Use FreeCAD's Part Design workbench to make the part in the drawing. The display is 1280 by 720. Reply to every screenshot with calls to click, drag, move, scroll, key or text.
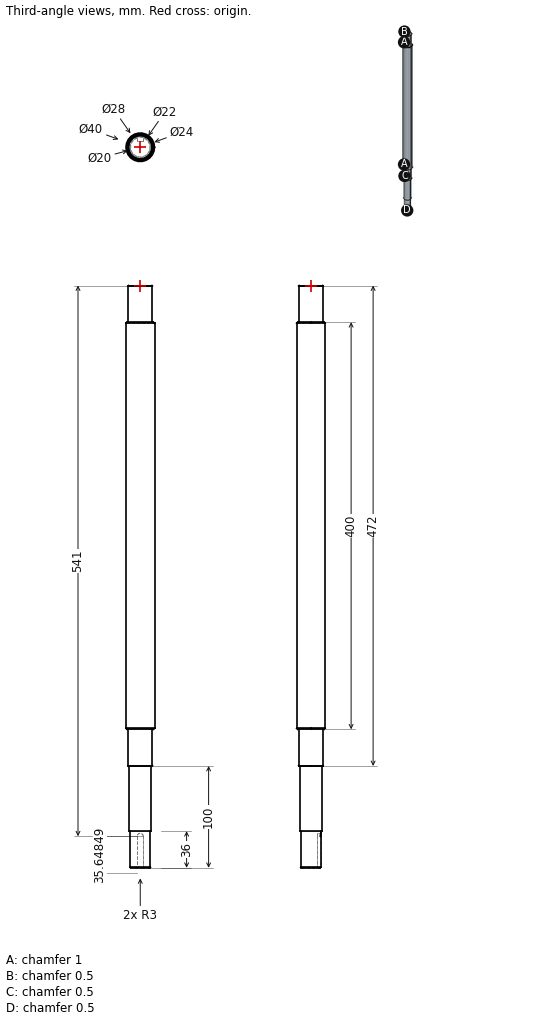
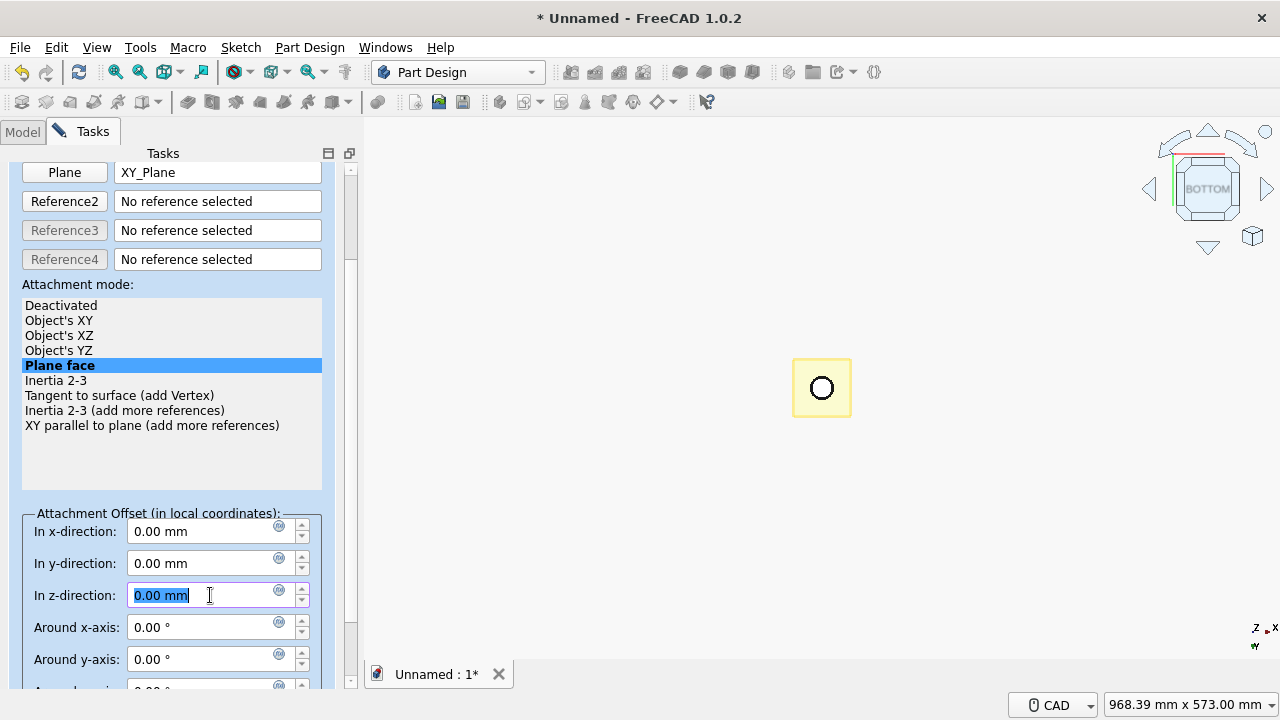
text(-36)
key(Tab)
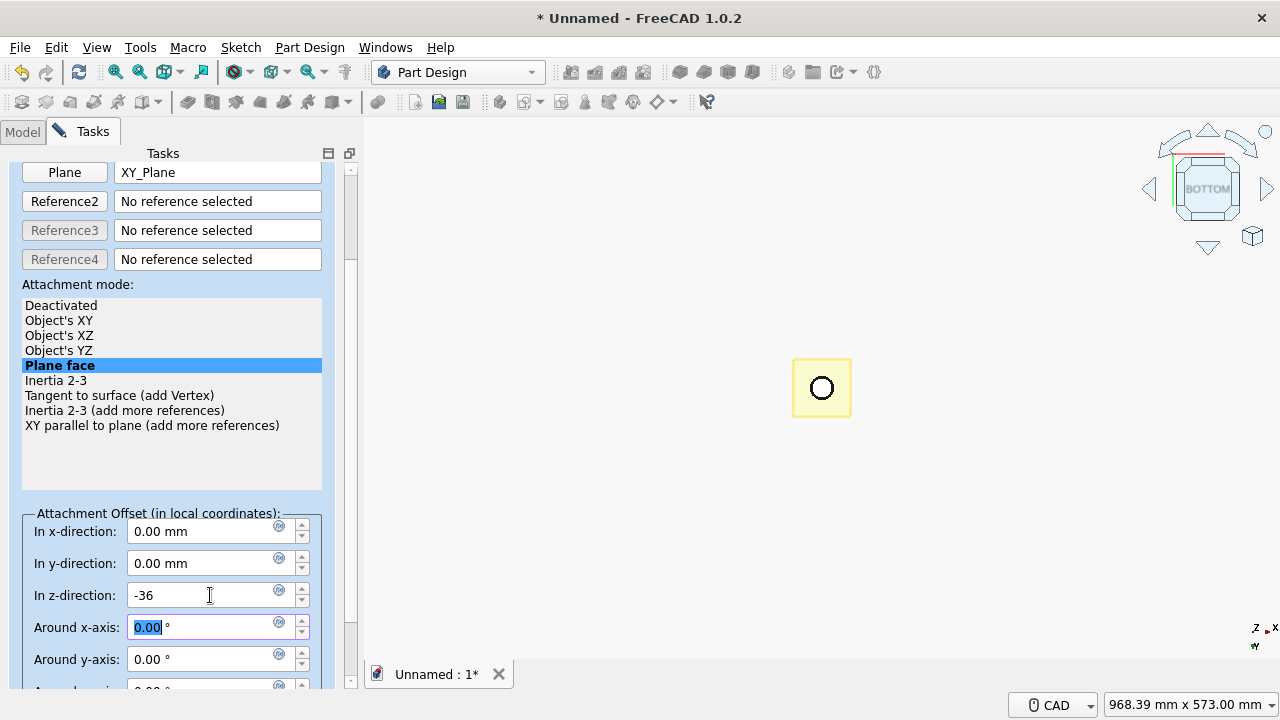
scroll(351, 426, up, 3)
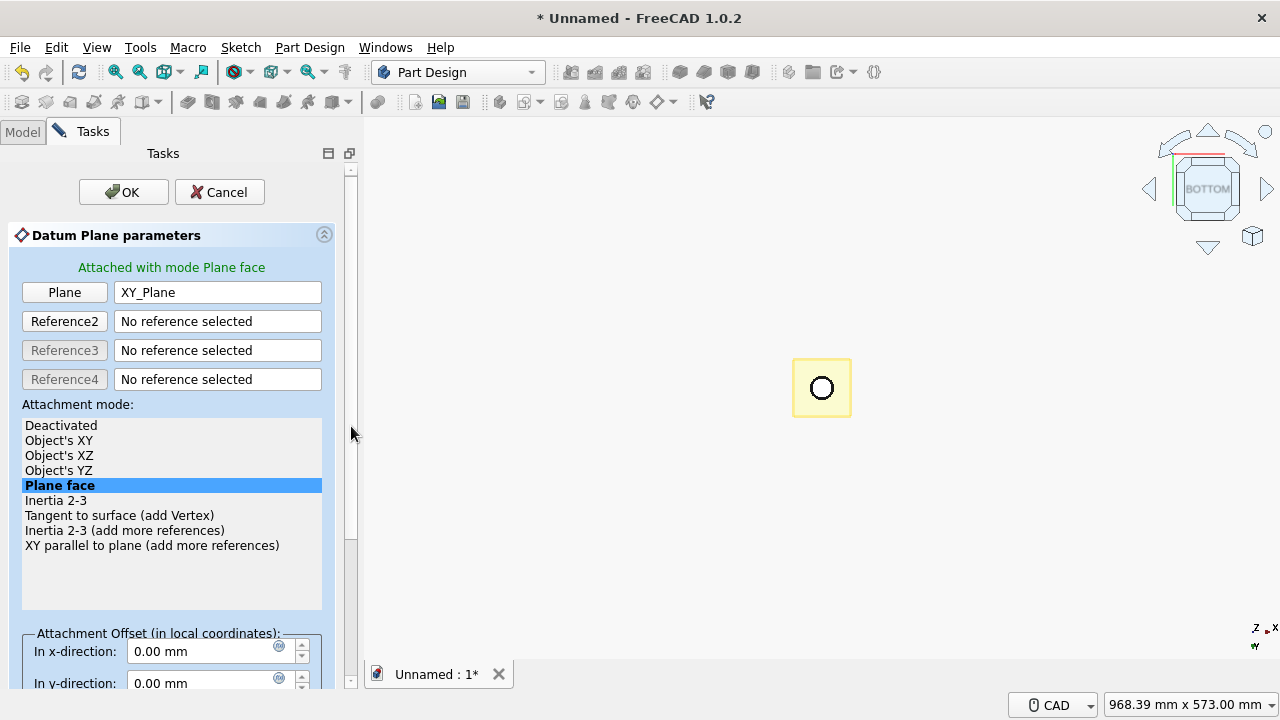
click(124, 192)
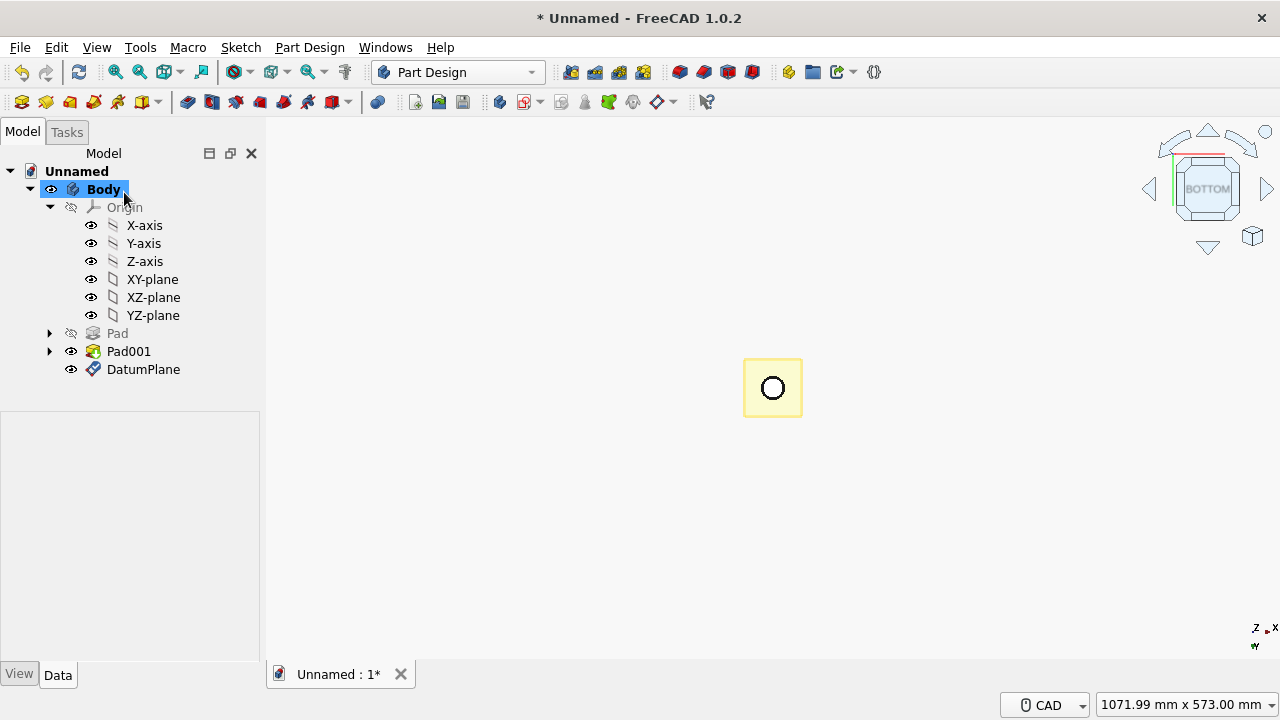
click(116, 369)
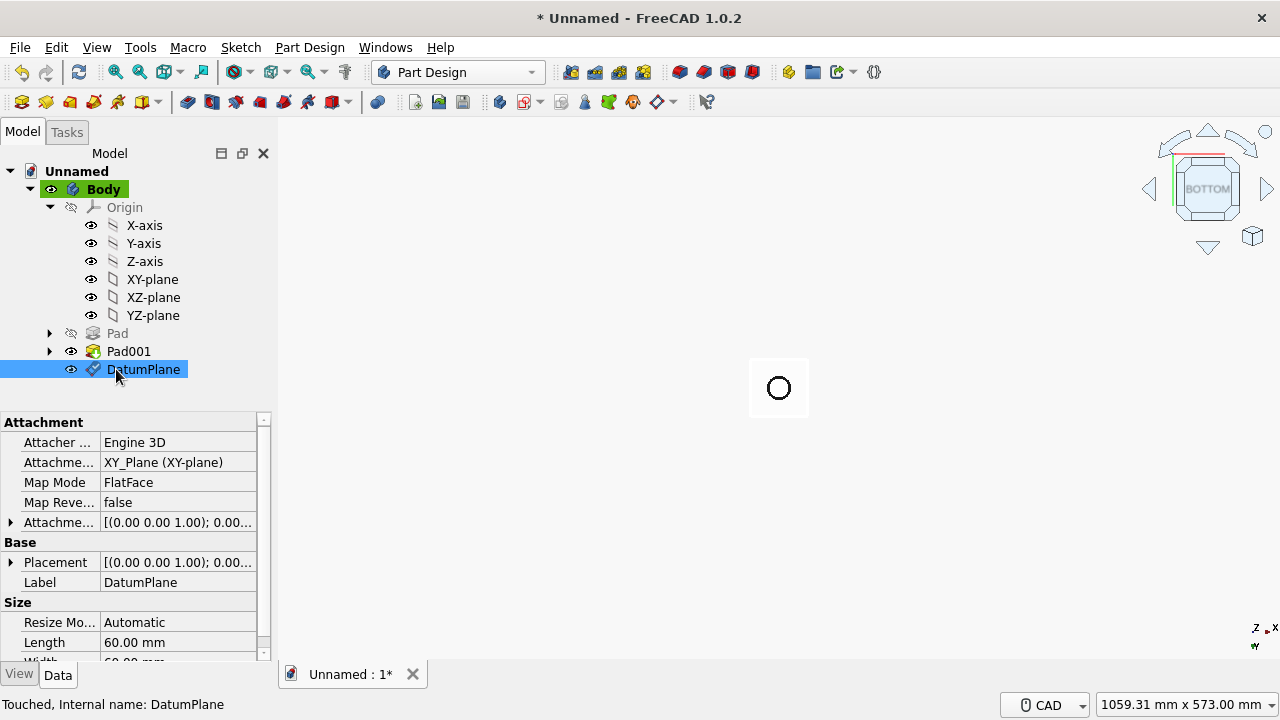
click(524, 102)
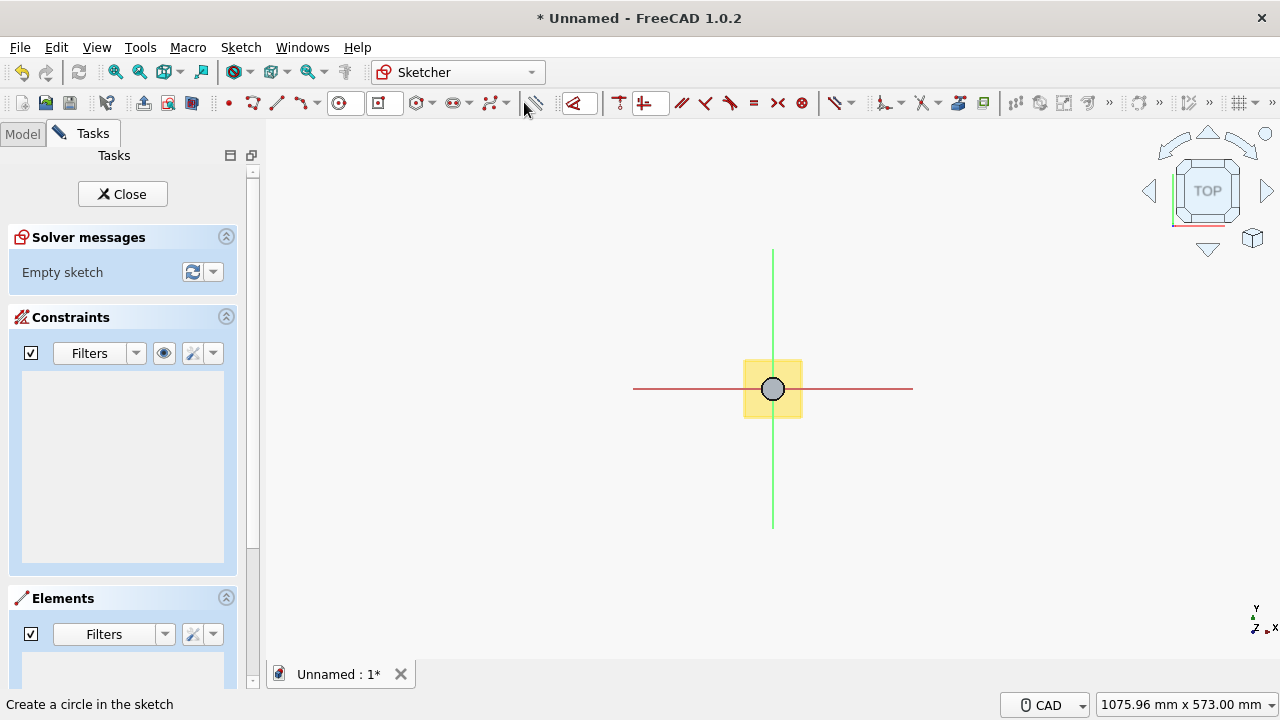
click(192, 104)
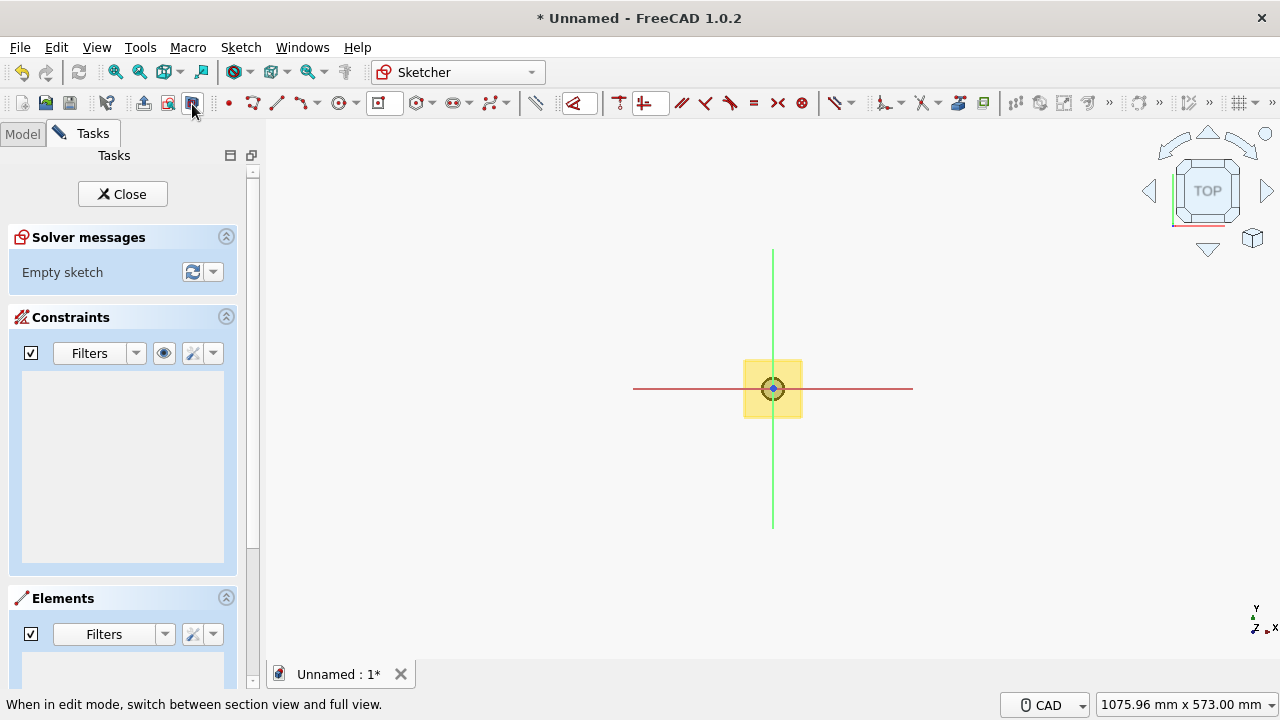
scroll(778, 389, up, 13)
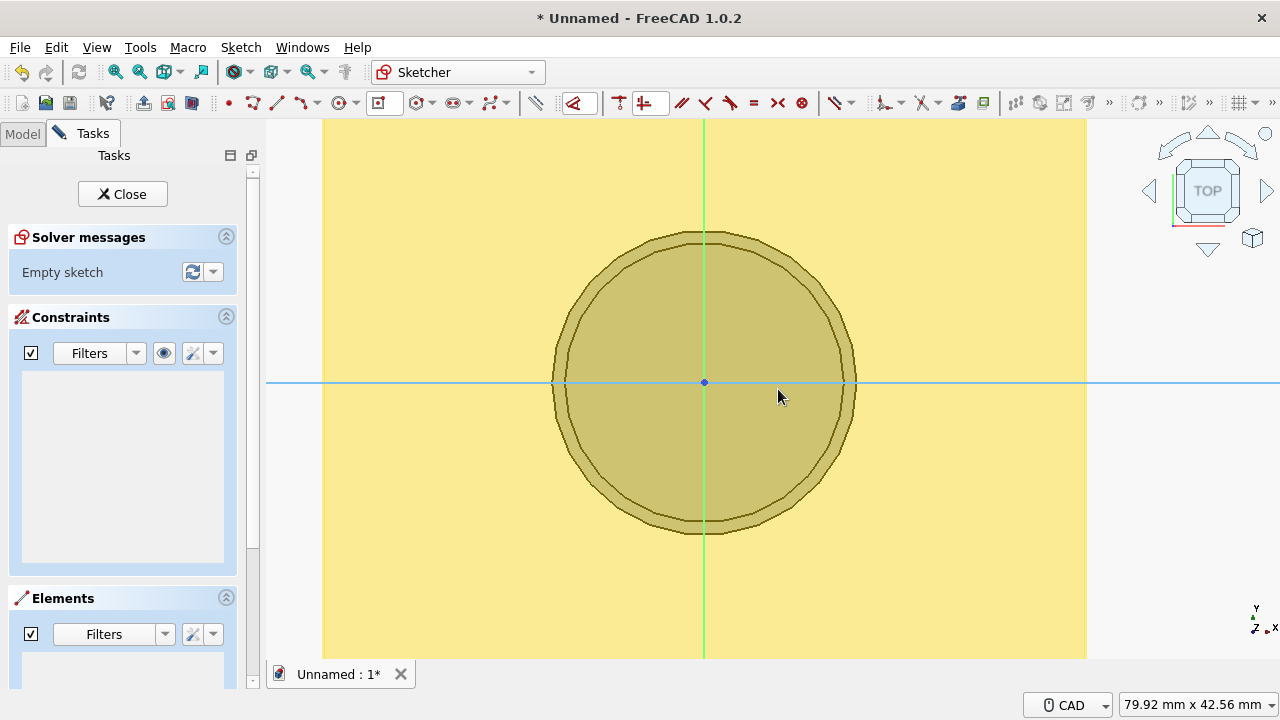
click(340, 104)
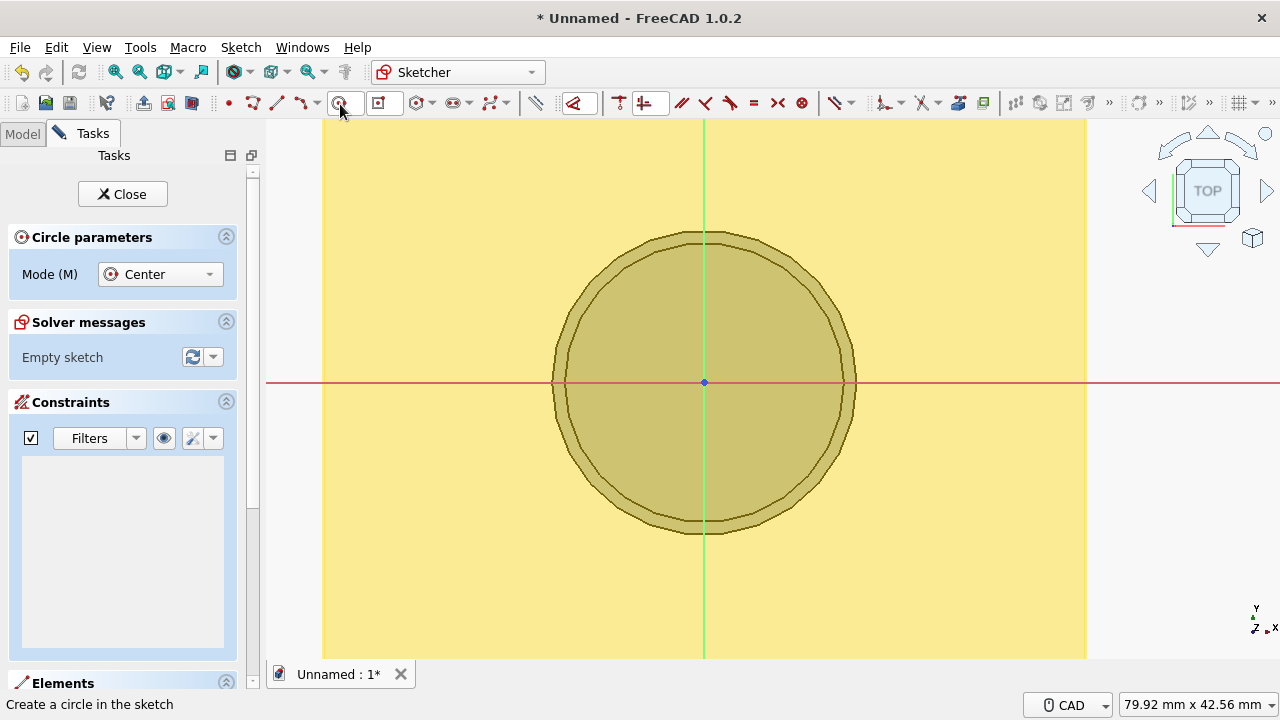
click(704, 383)
move(830, 257)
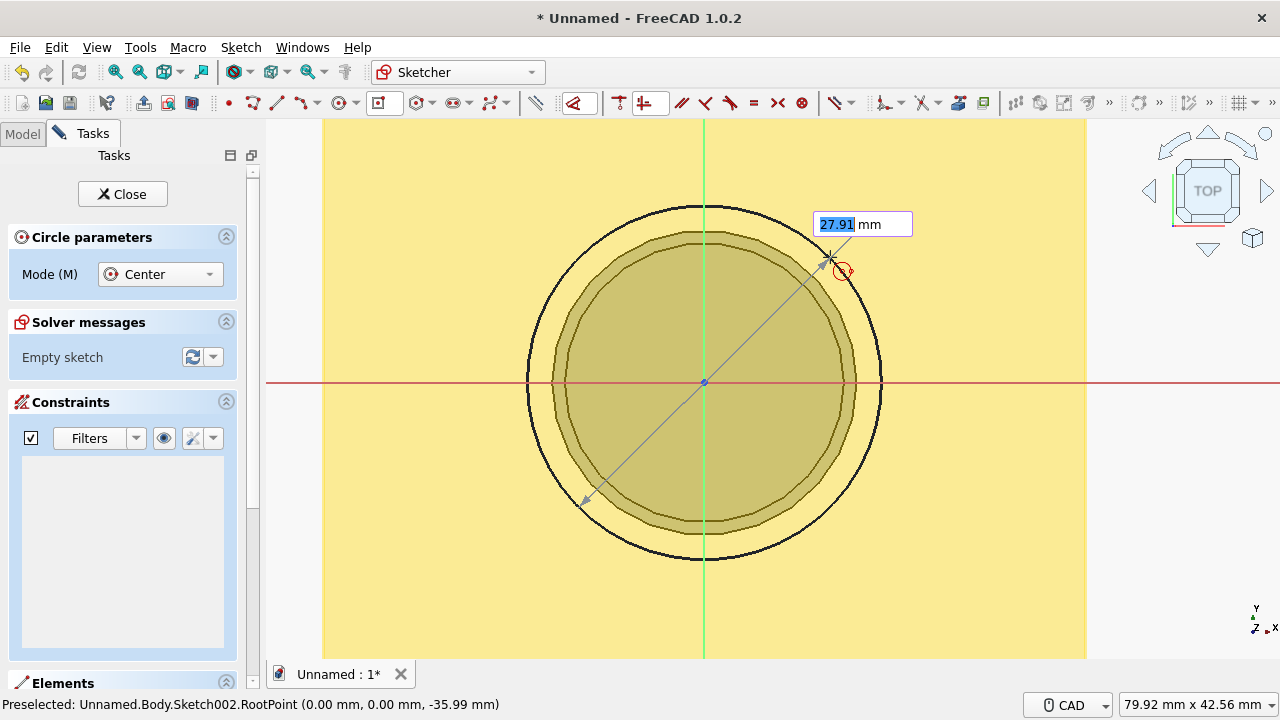
text(28)
key(Return)
key(Escape)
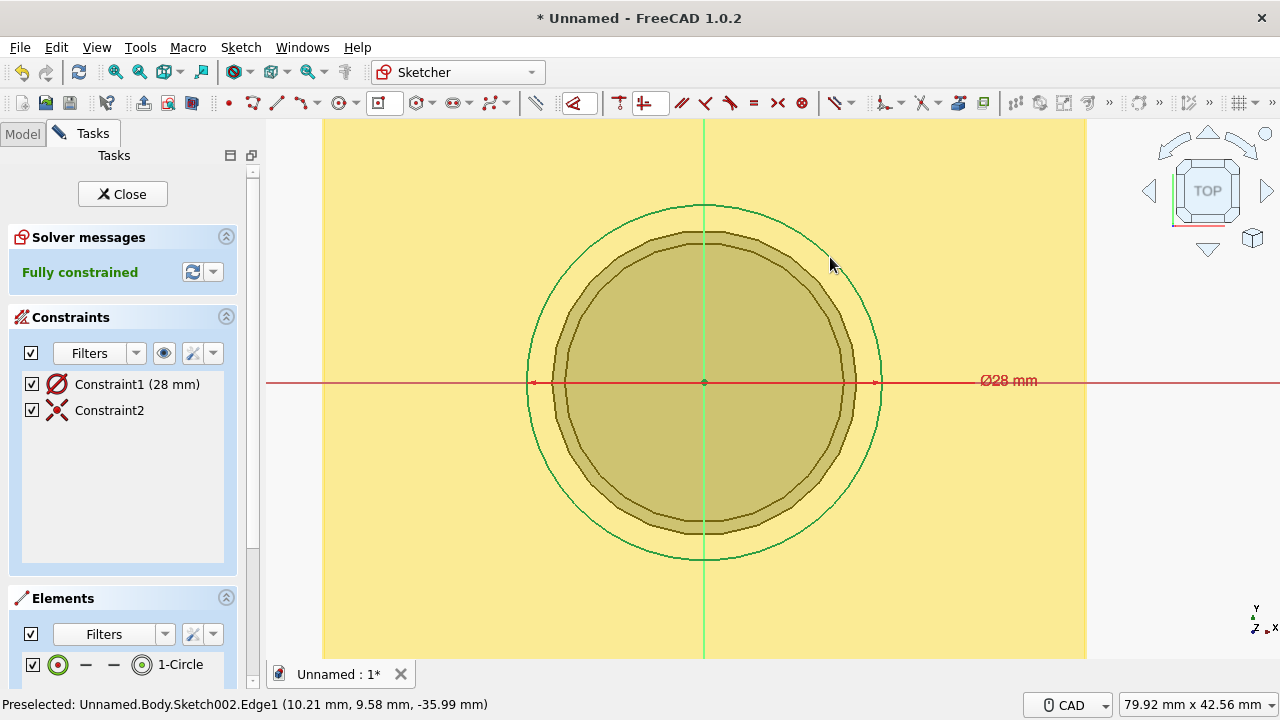
click(123, 194)